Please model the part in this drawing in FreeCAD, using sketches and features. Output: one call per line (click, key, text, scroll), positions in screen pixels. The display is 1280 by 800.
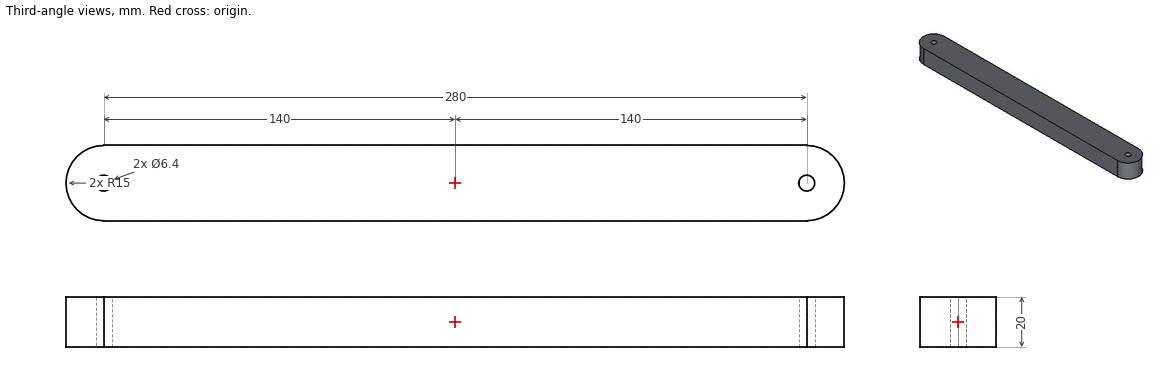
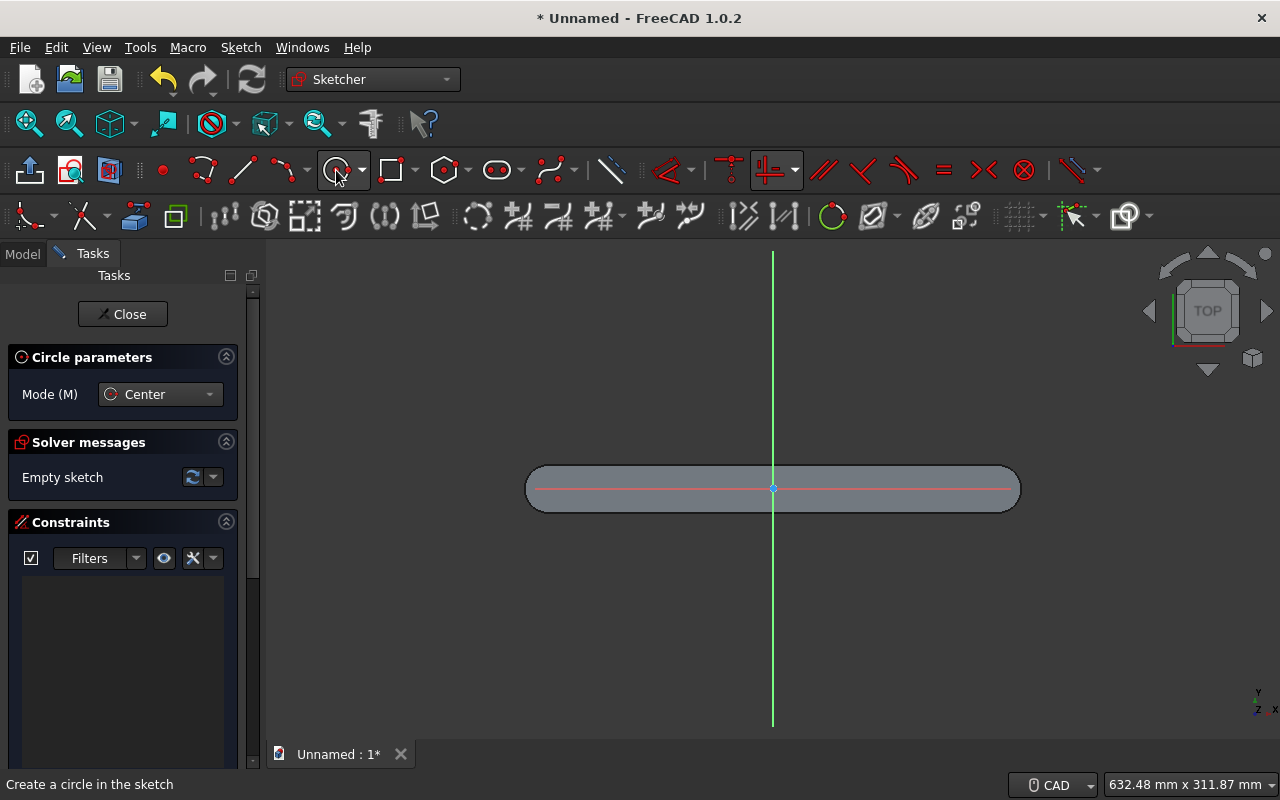
scroll(549, 489, up, 8)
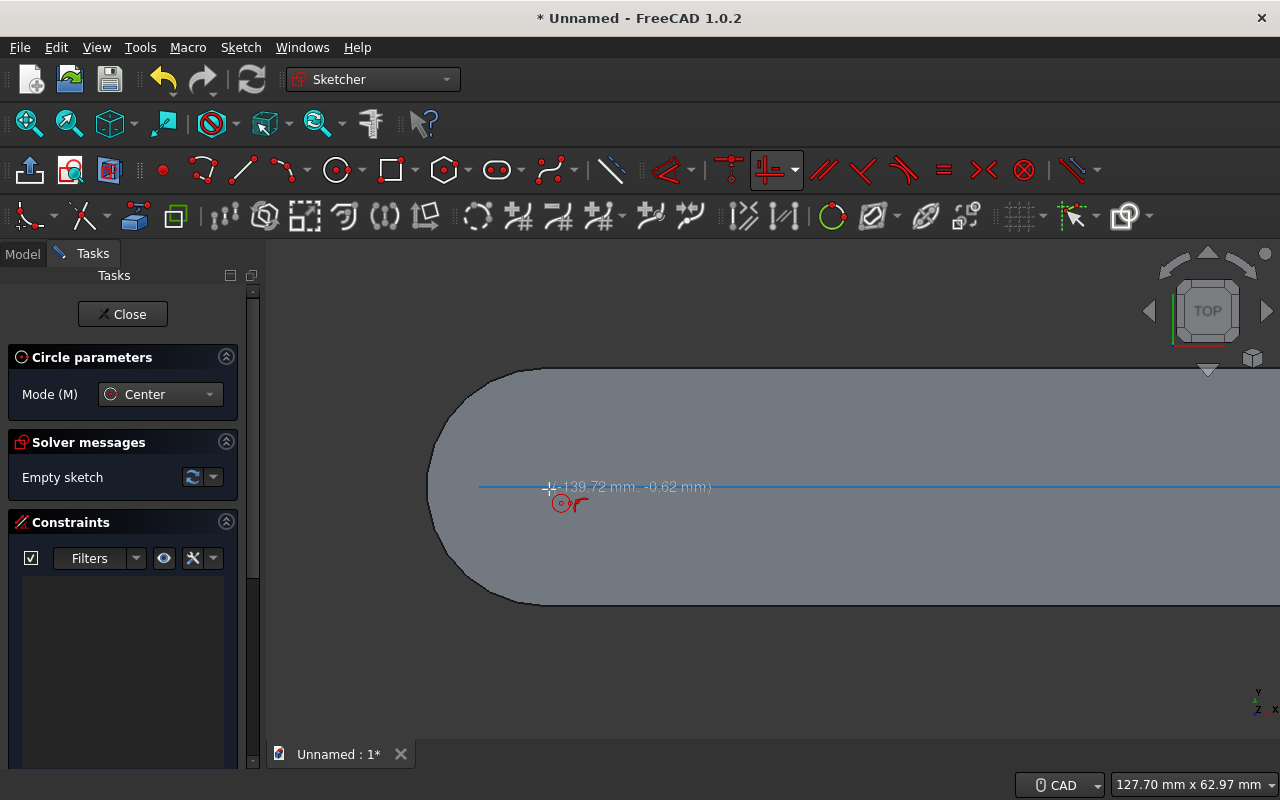
scroll(393, 490, down, 7)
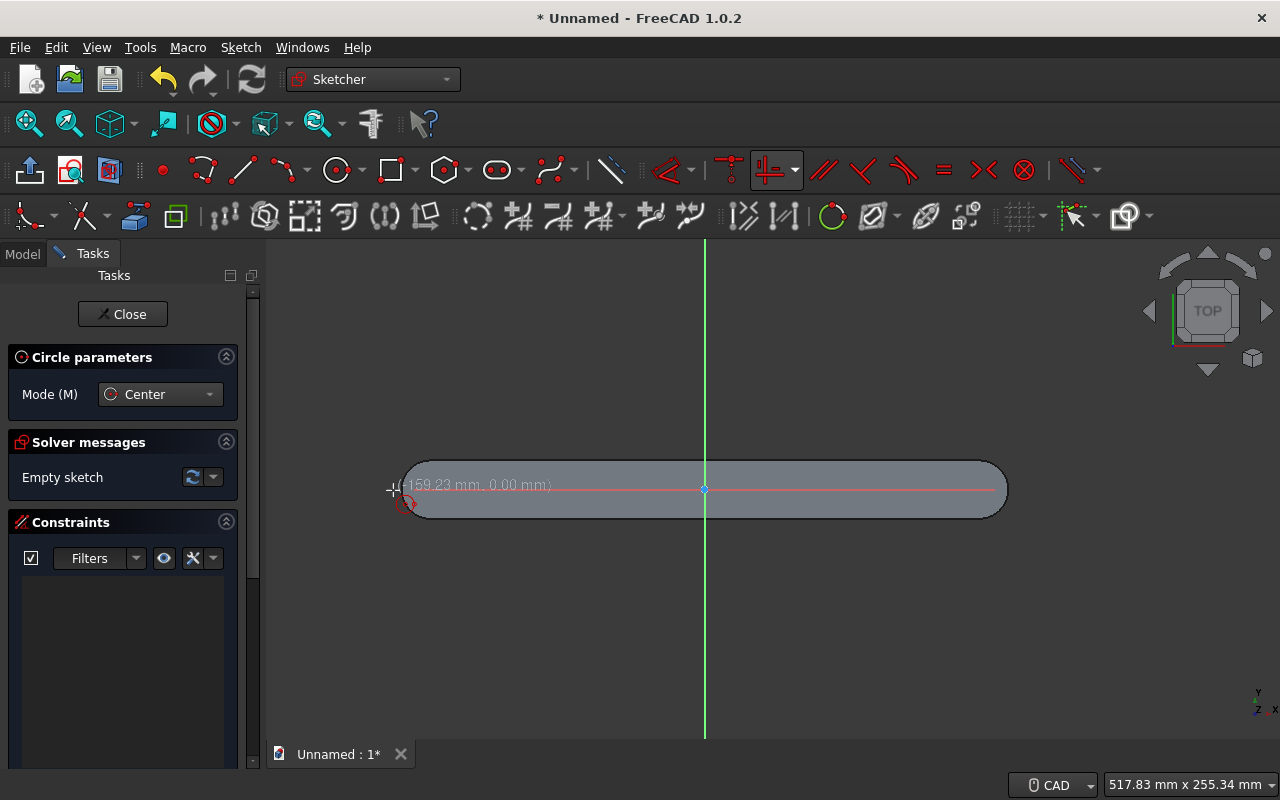
click(431, 490)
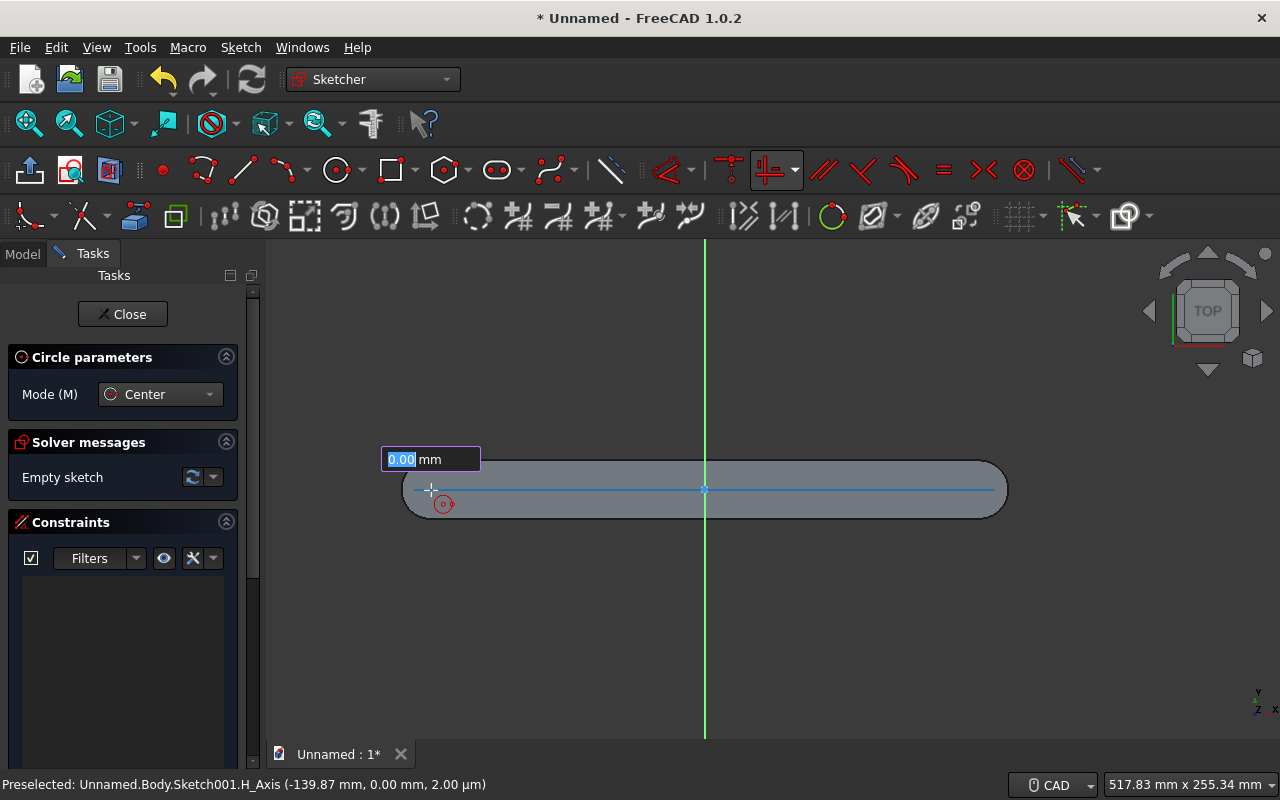
scroll(429, 496, up, 5)
move(428, 494)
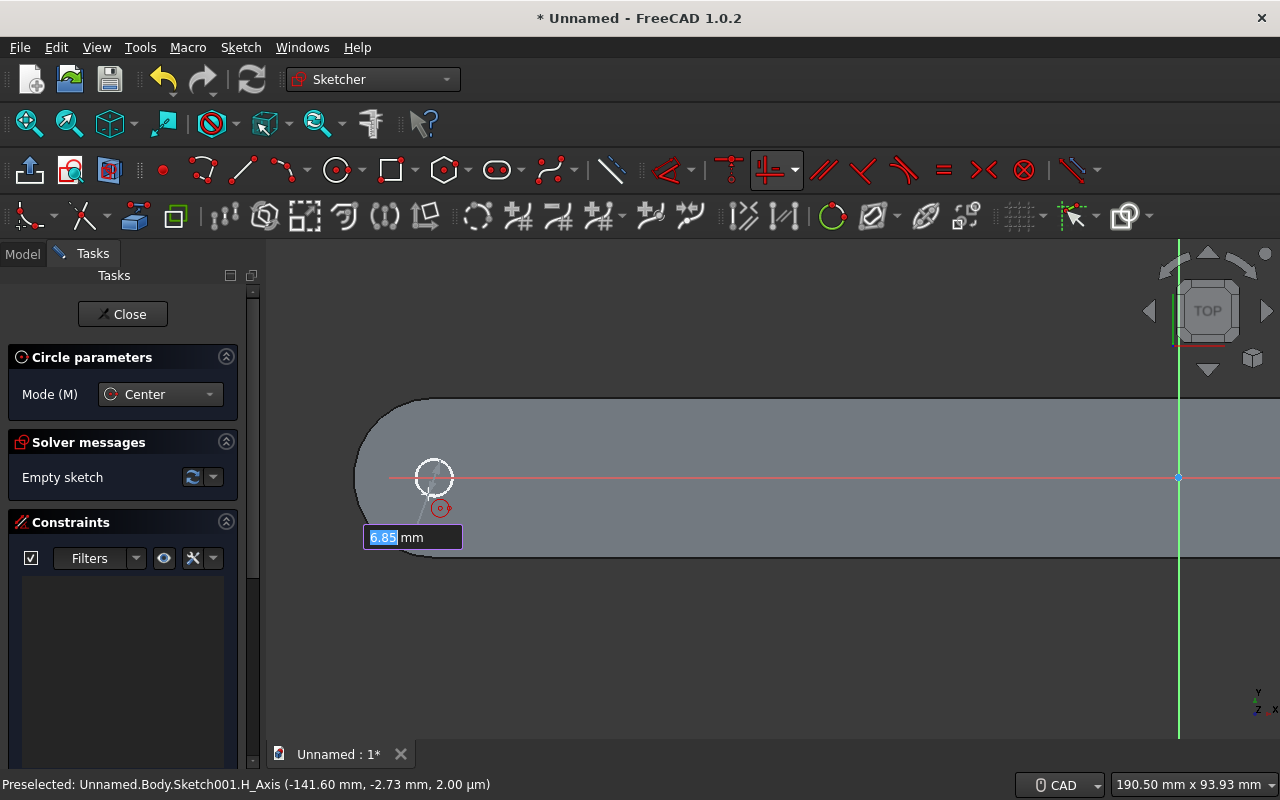
text(6.4)
key(Return)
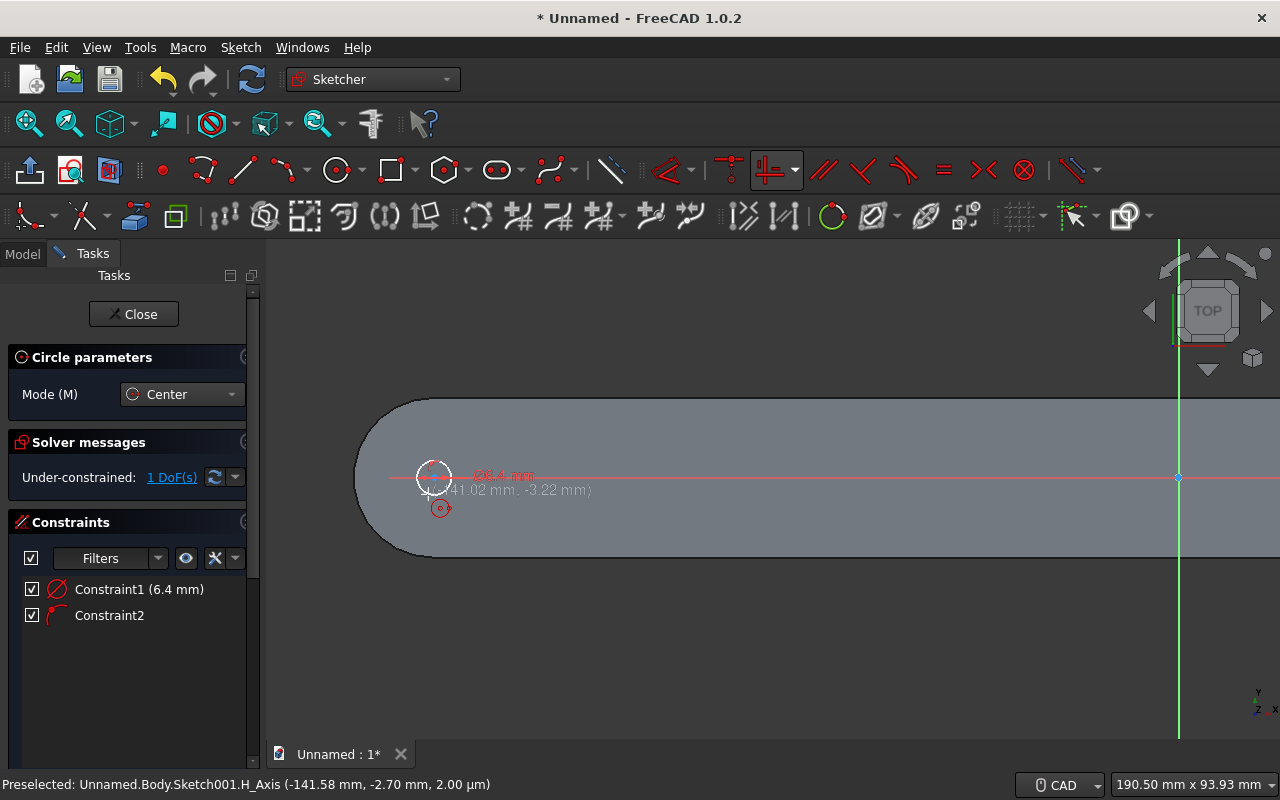
scroll(429, 495, down, 5)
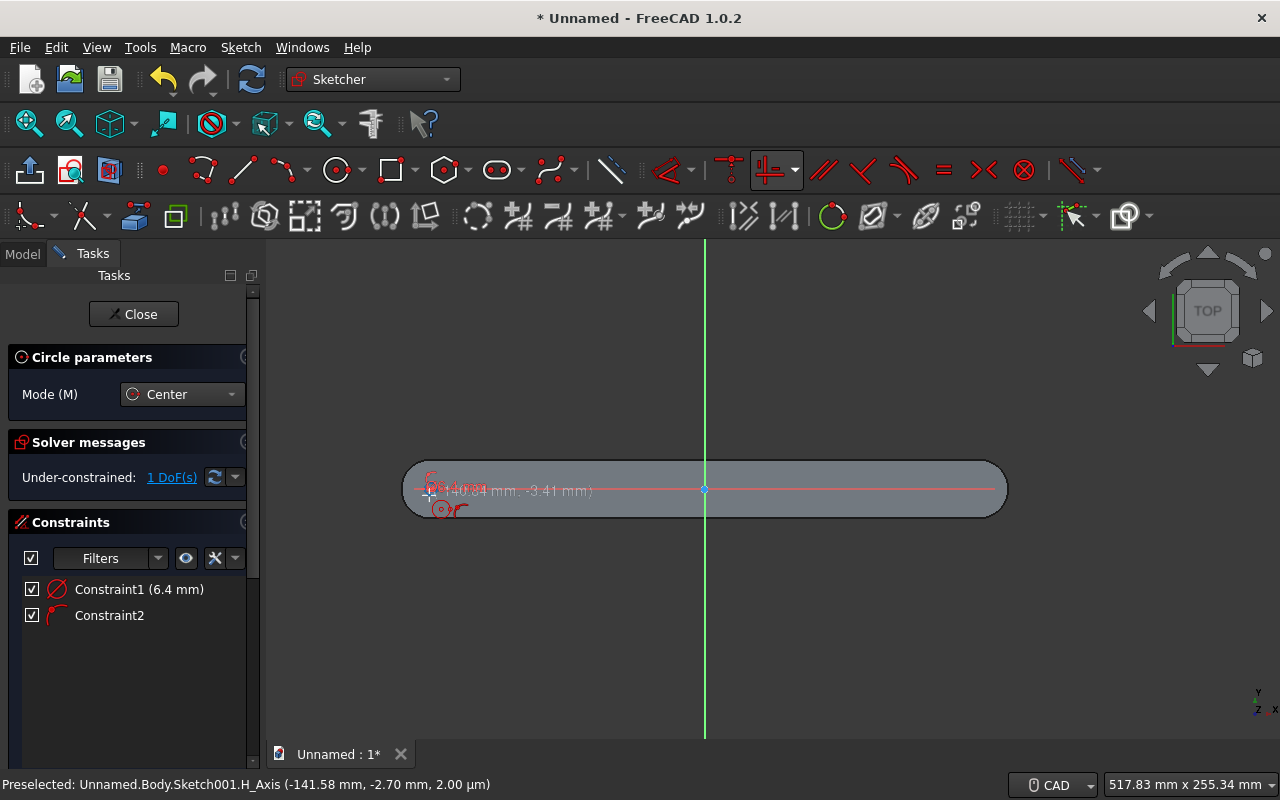
scroll(979, 489, up, 7)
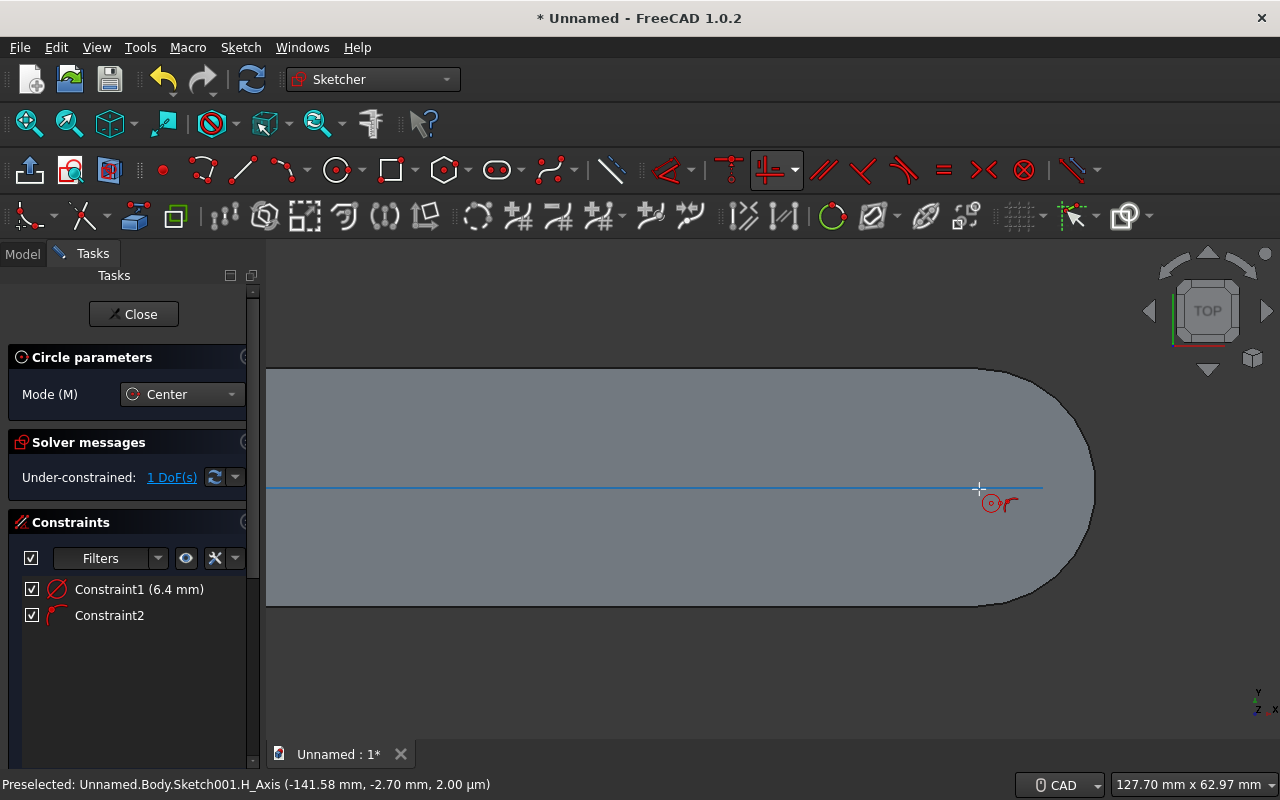
scroll(979, 489, down, 7)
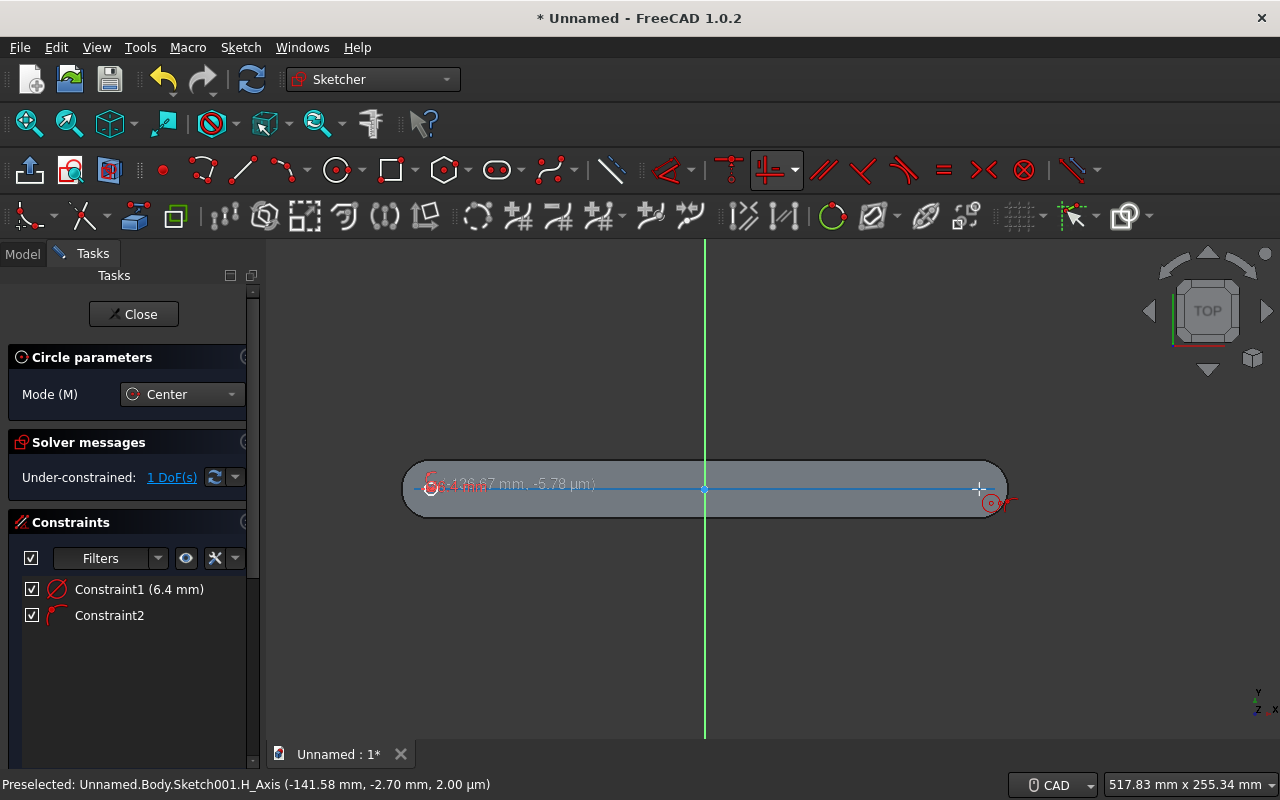
click(979, 489)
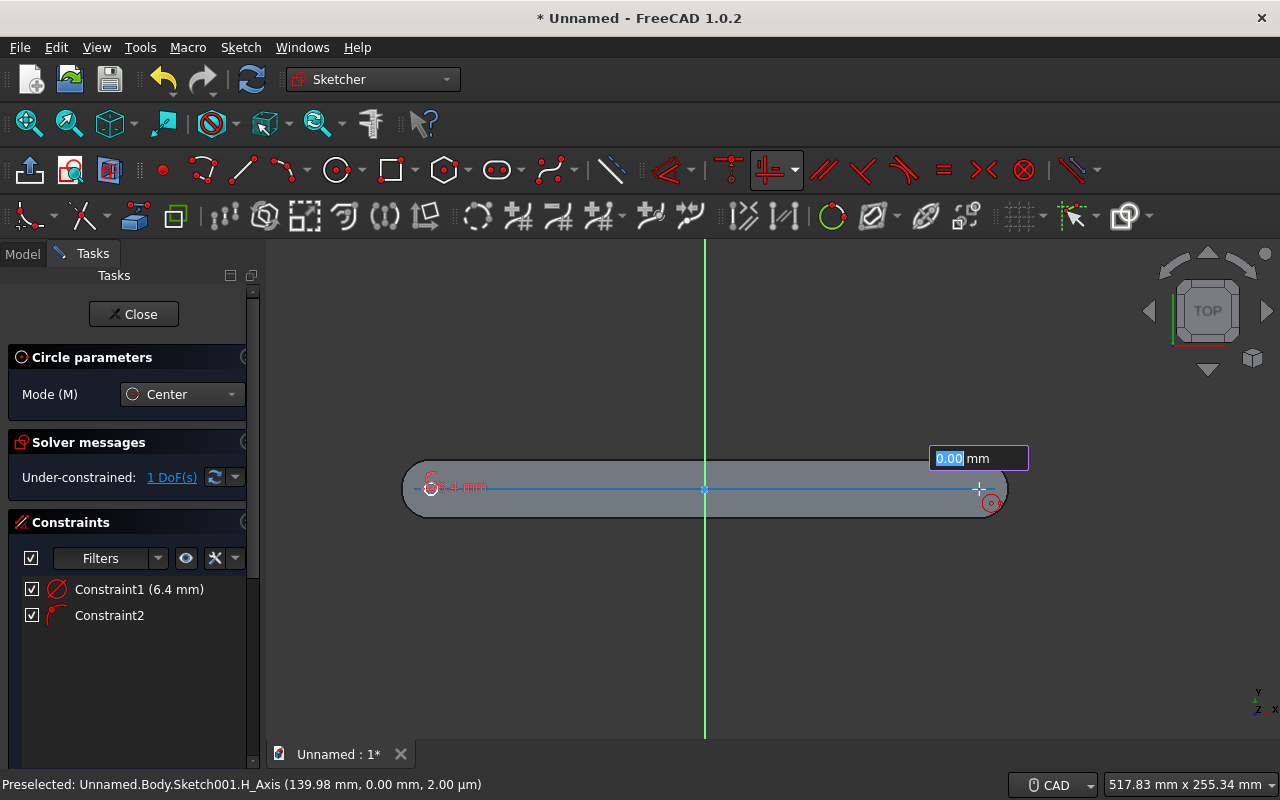
scroll(977, 495, up, 5)
move(975, 494)